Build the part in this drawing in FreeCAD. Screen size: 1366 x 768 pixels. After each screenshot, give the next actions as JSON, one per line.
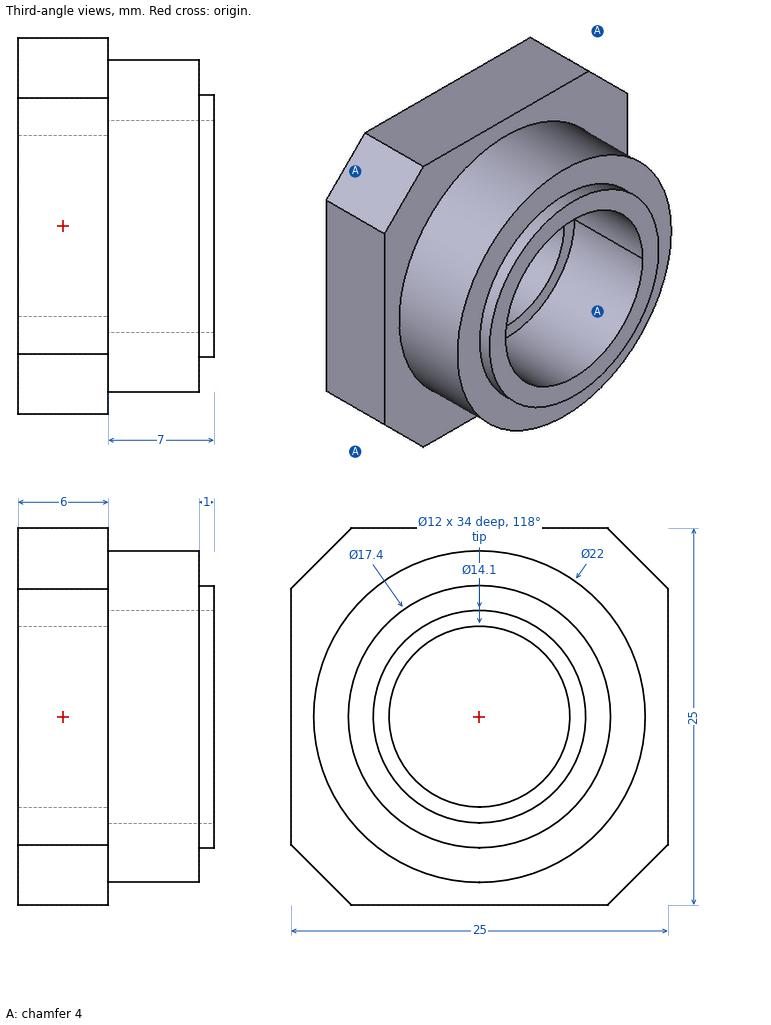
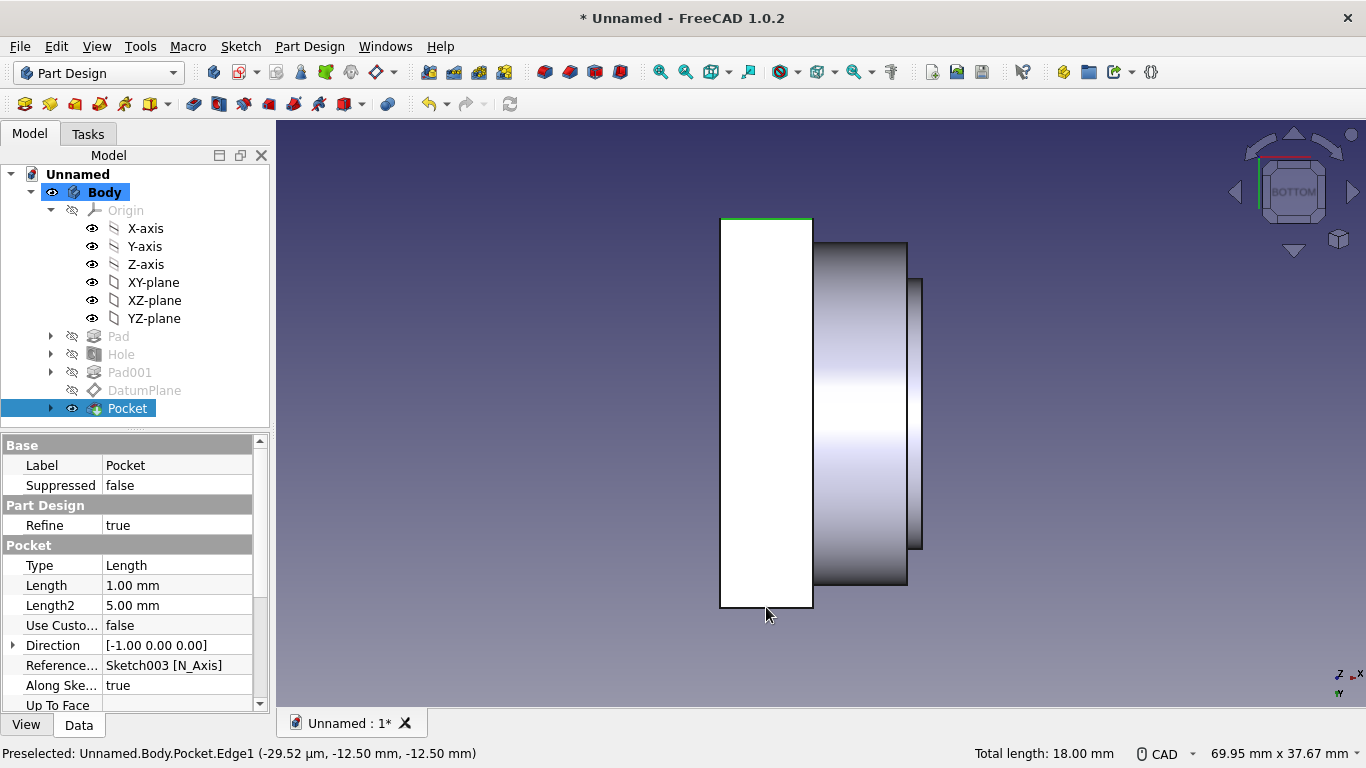
{"action": "left_click", "coordinate": [766, 607], "text": "ctrl"}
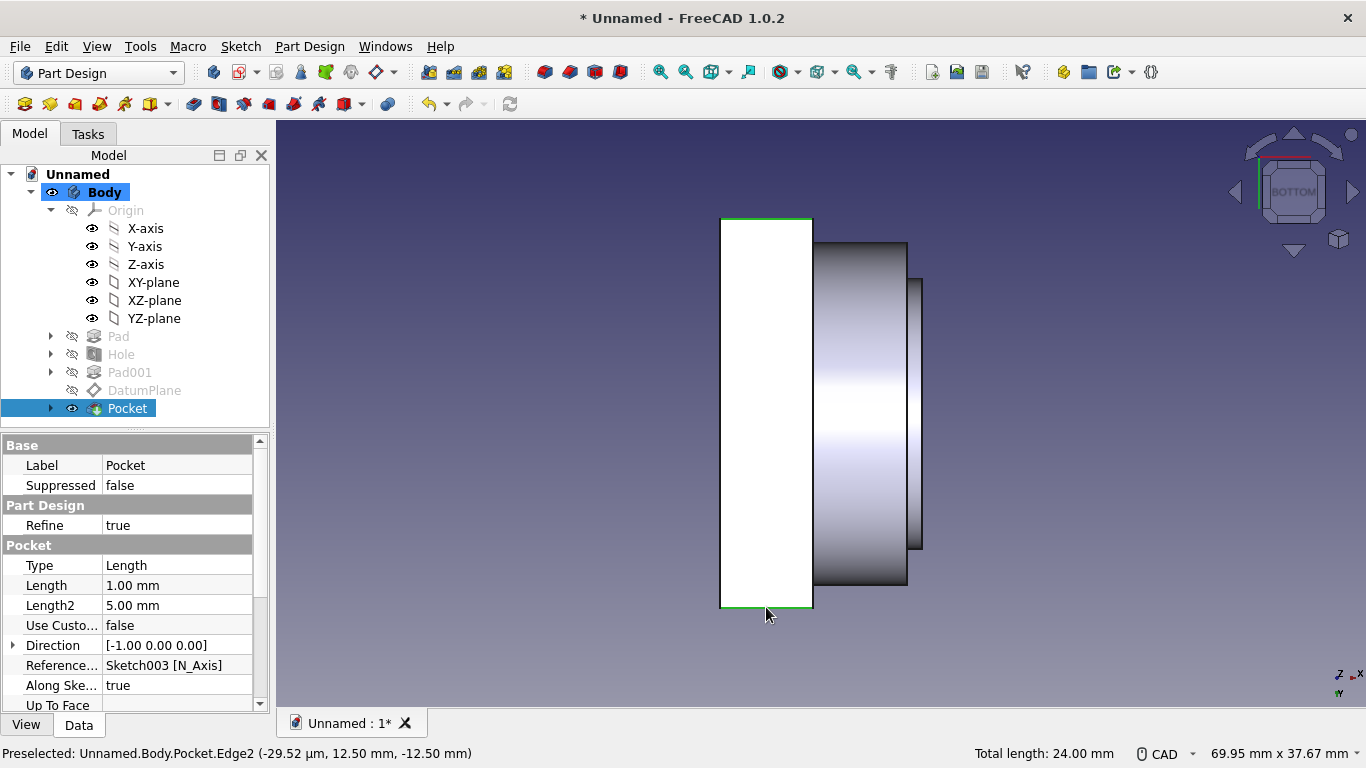
{"action": "left_click", "coordinate": [570, 72]}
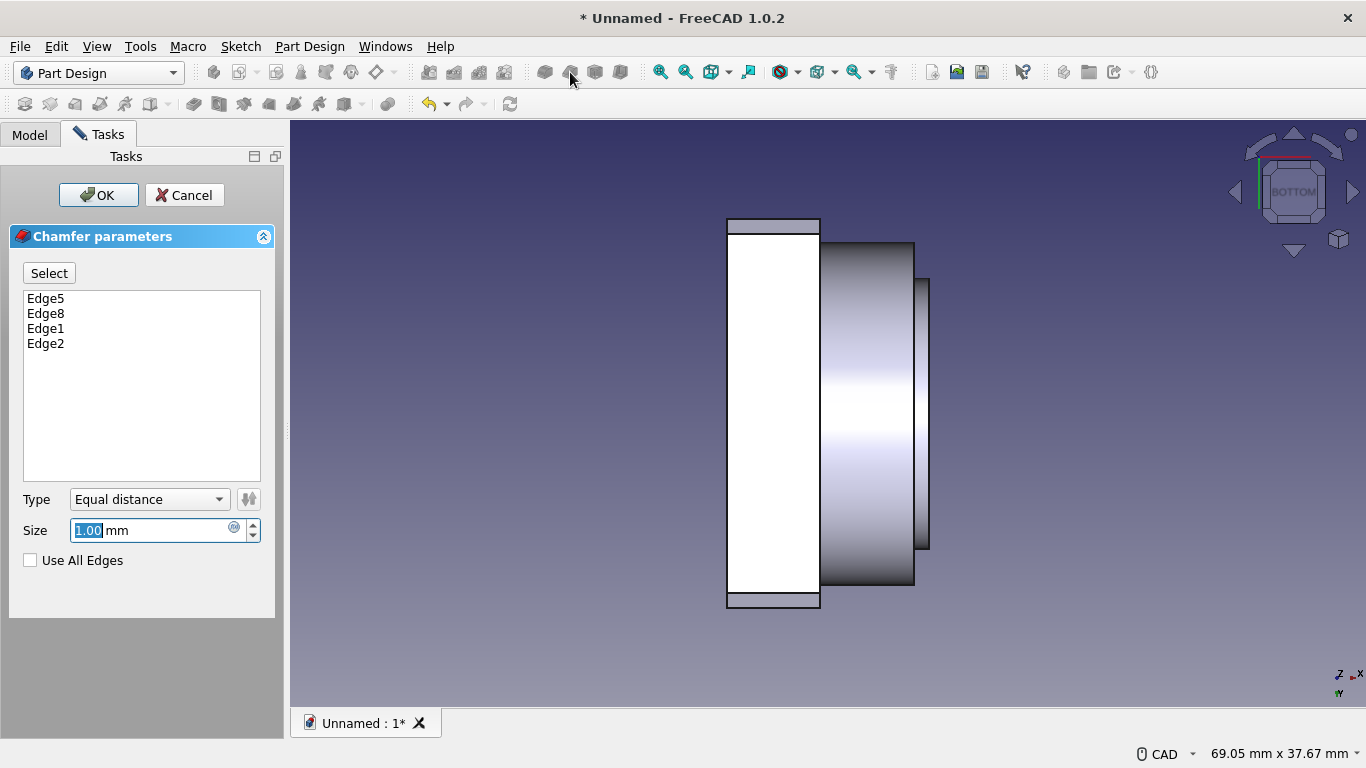
{"action": "type", "text": "4"}
{"action": "key", "text": "Tab"}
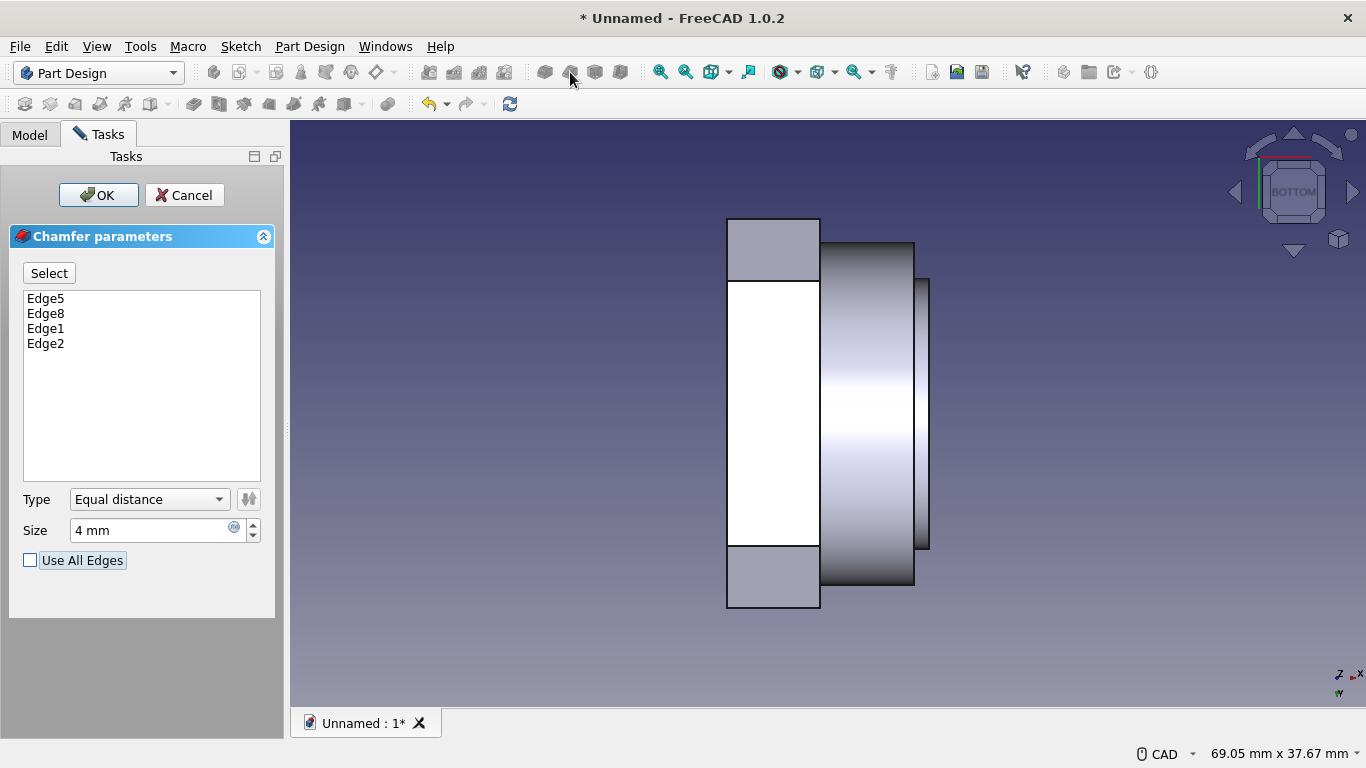
{"action": "left_click", "coordinate": [99, 195]}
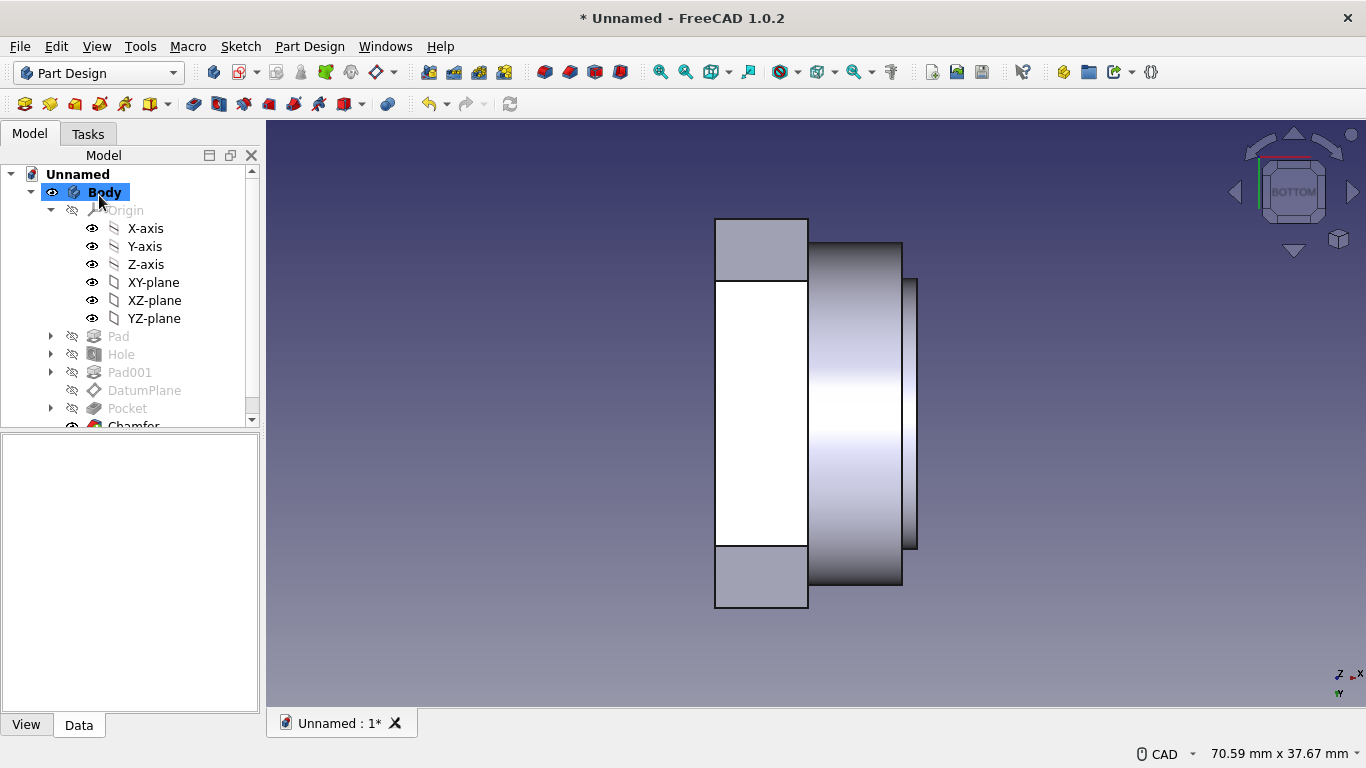
{"action": "key", "text": "0"}